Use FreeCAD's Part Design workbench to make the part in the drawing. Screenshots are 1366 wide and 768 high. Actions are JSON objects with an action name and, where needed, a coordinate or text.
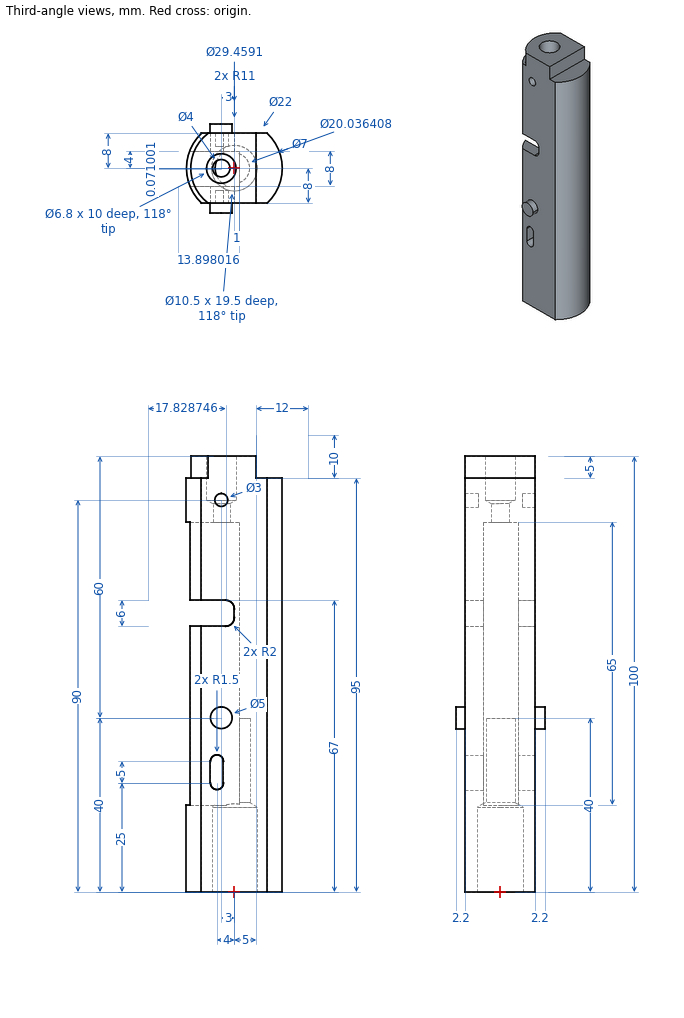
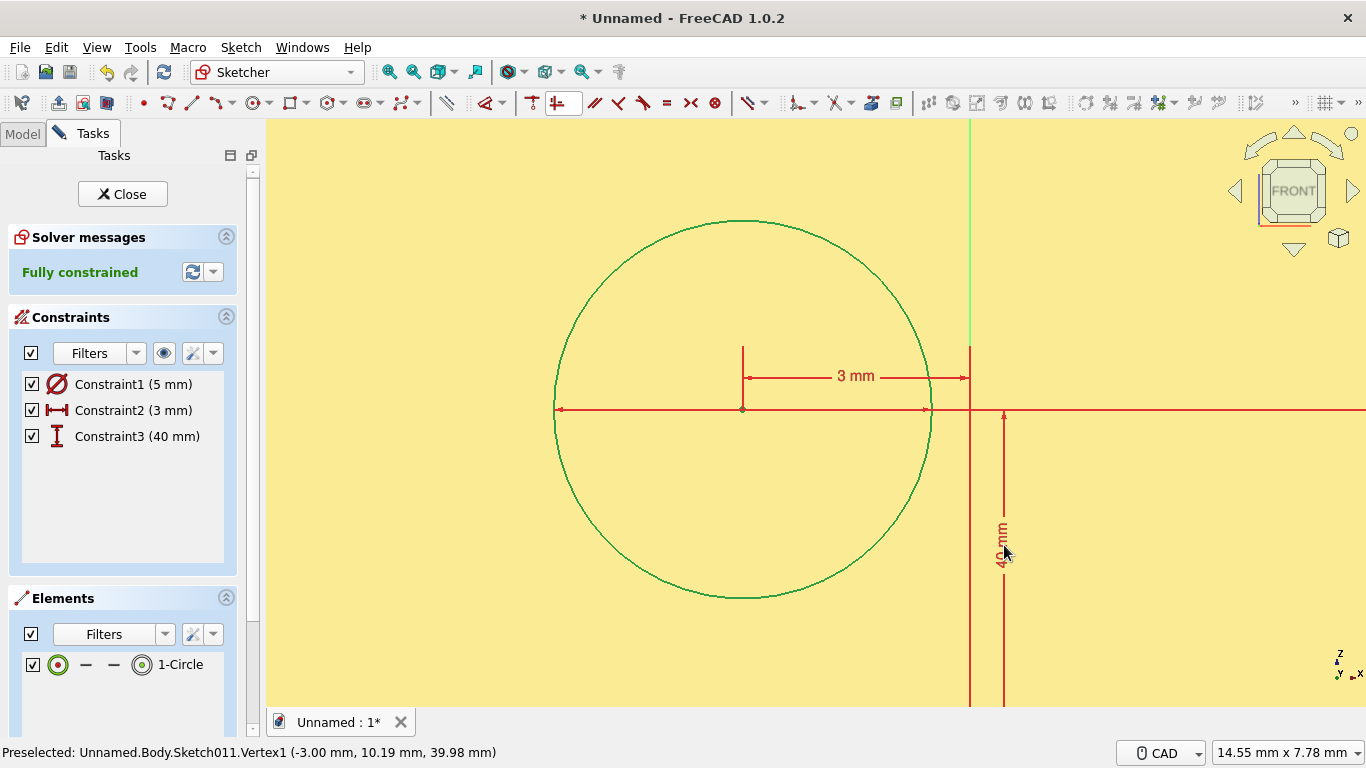
{"action": "left_click", "coordinate": [123, 194]}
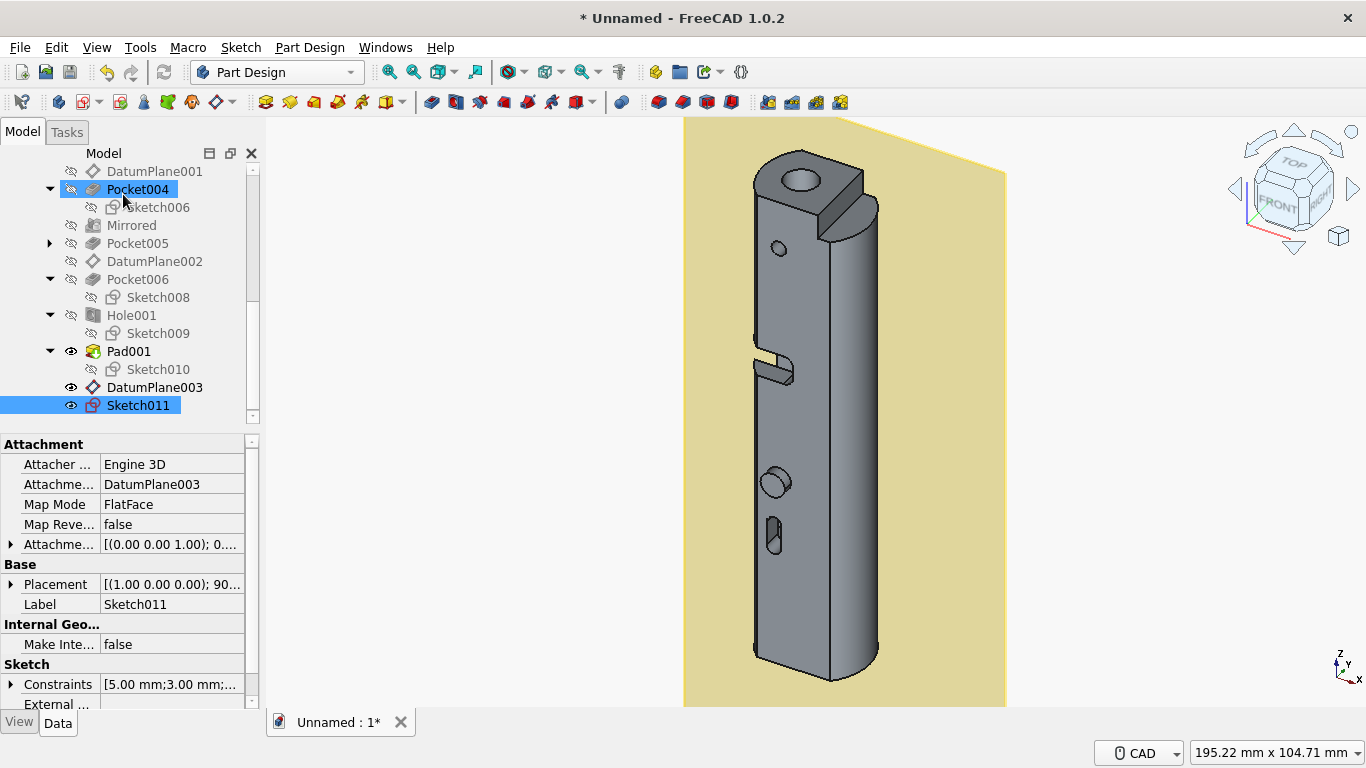
{"action": "left_click", "coordinate": [266, 102]}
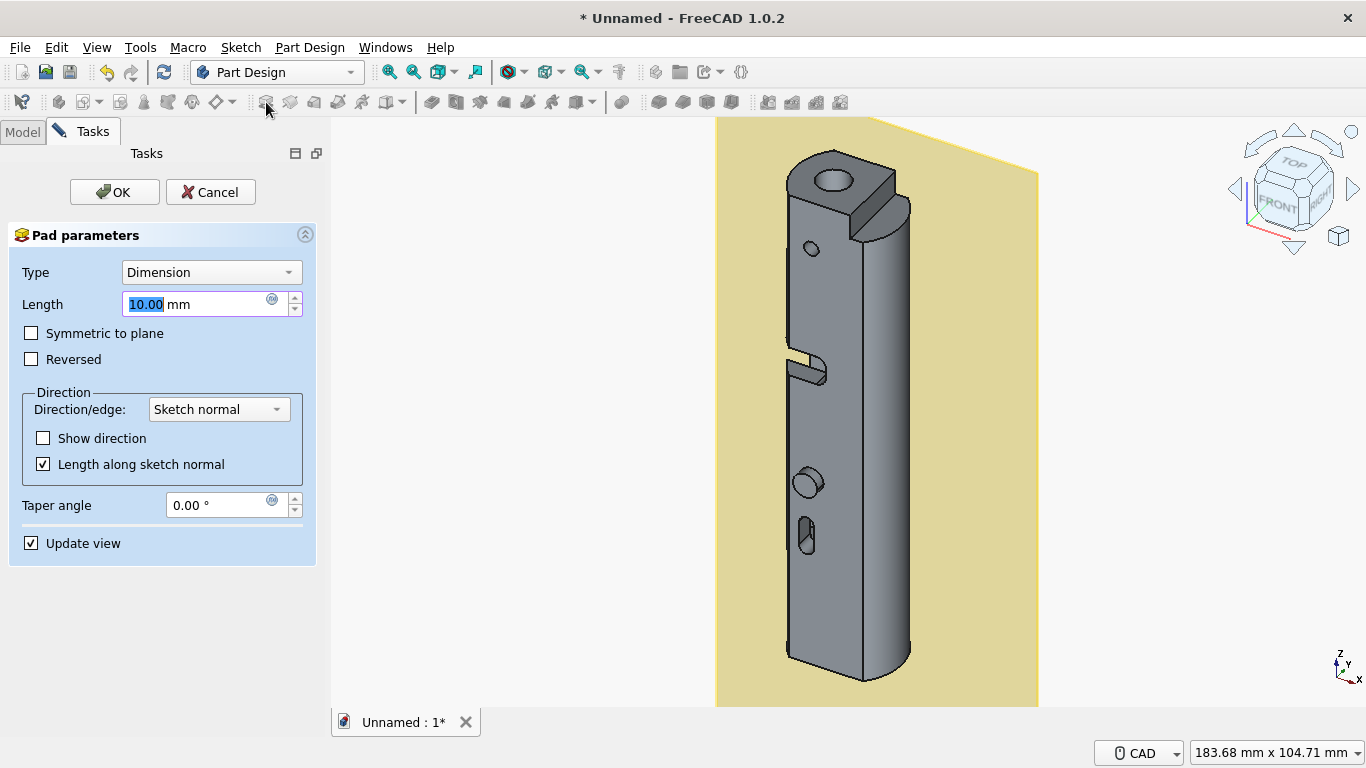
{"action": "type", "text": "2.2"}
{"action": "key", "text": "Tab"}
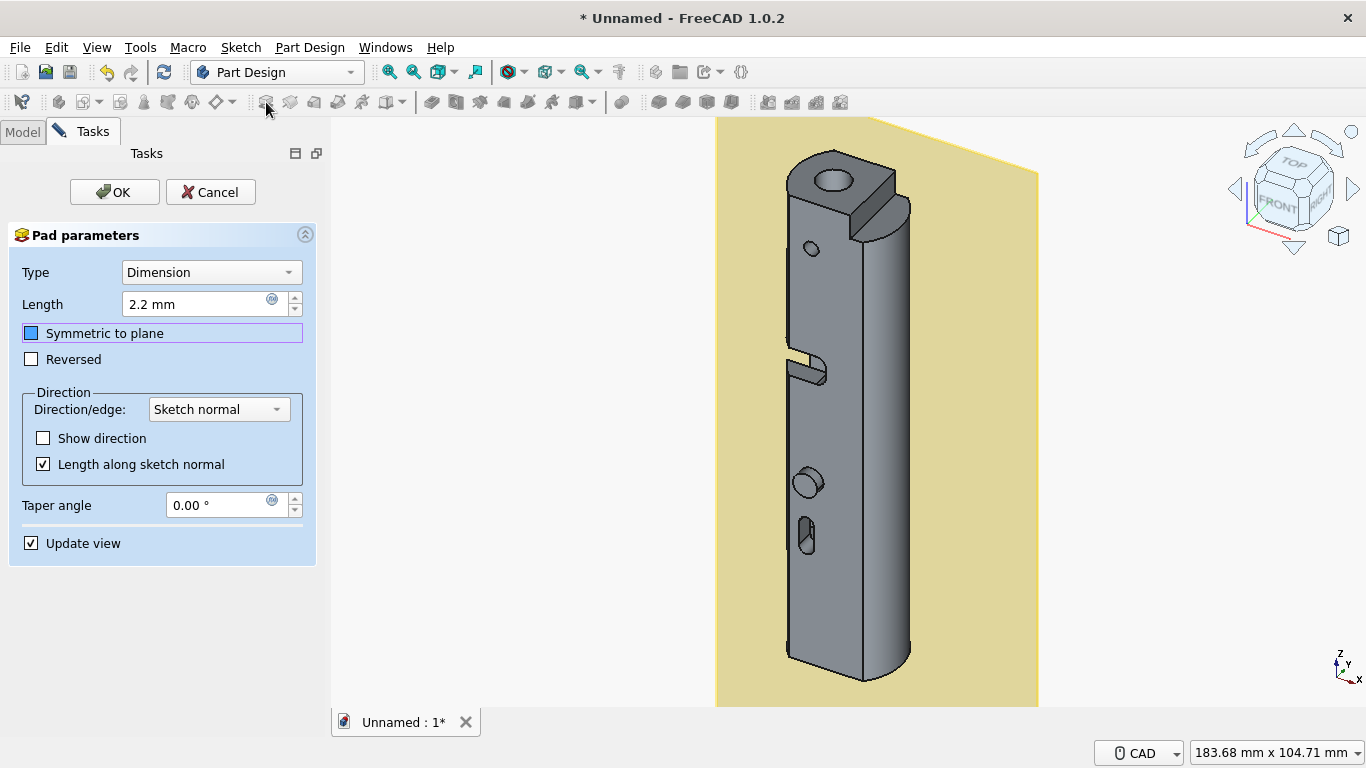
{"action": "left_click", "coordinate": [115, 192]}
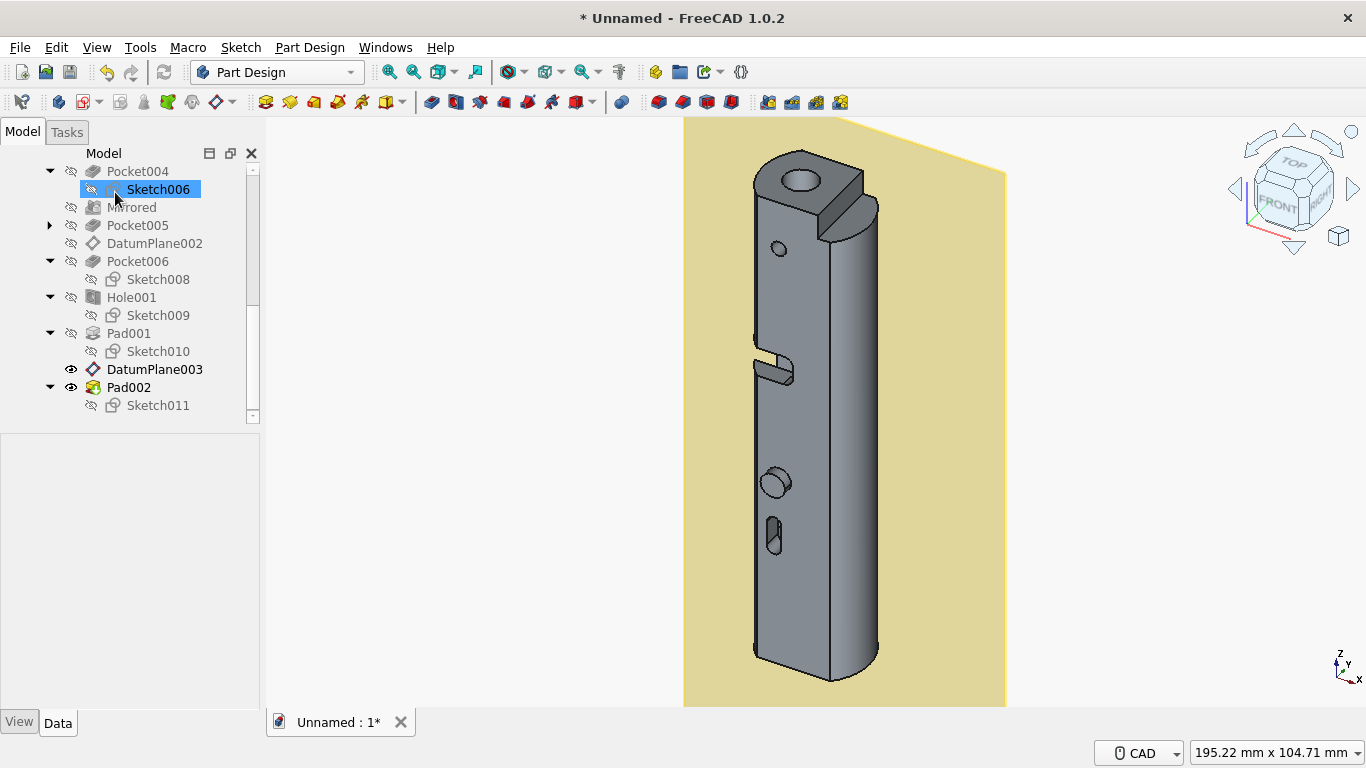
{"action": "left_click", "coordinate": [116, 369]}
{"action": "key", "text": "space"}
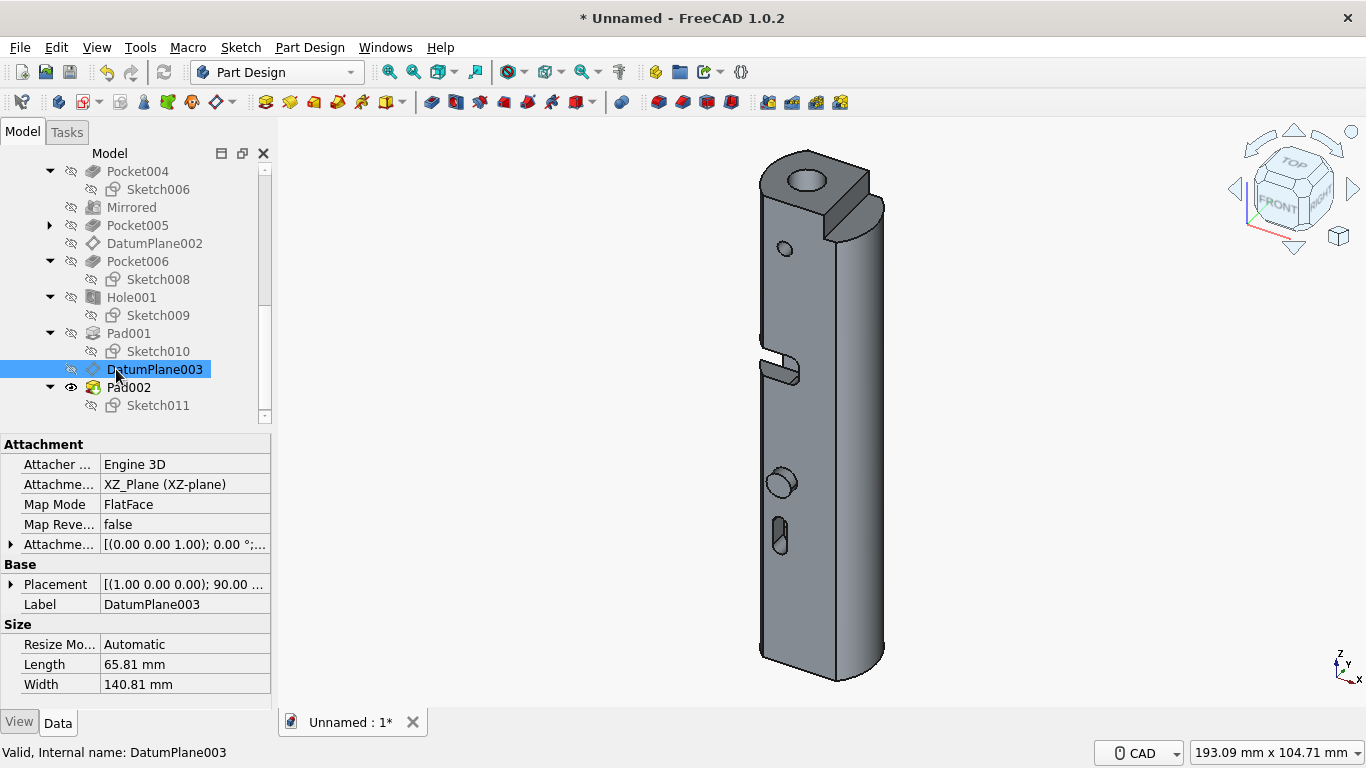
{"action": "left_click", "coordinate": [318, 667]}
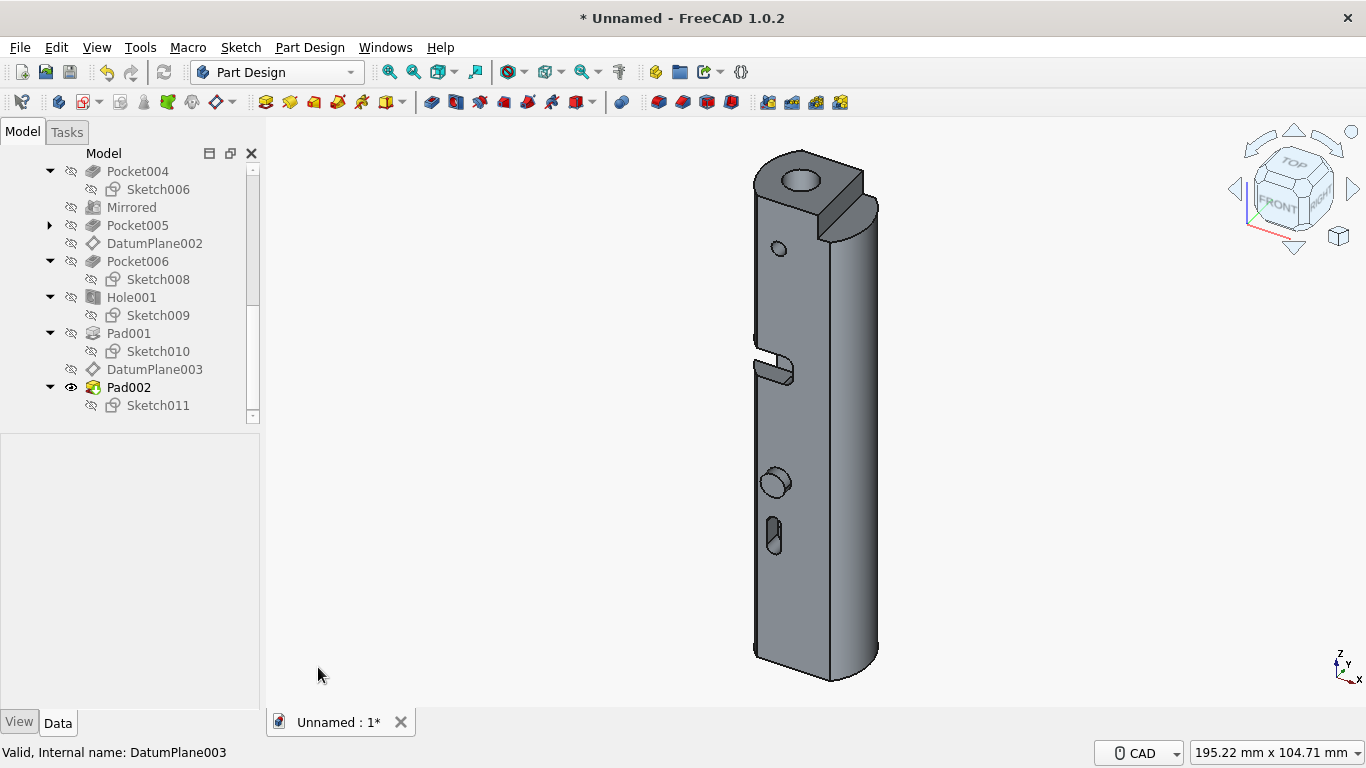
{"action": "left_click", "coordinate": [84, 102]}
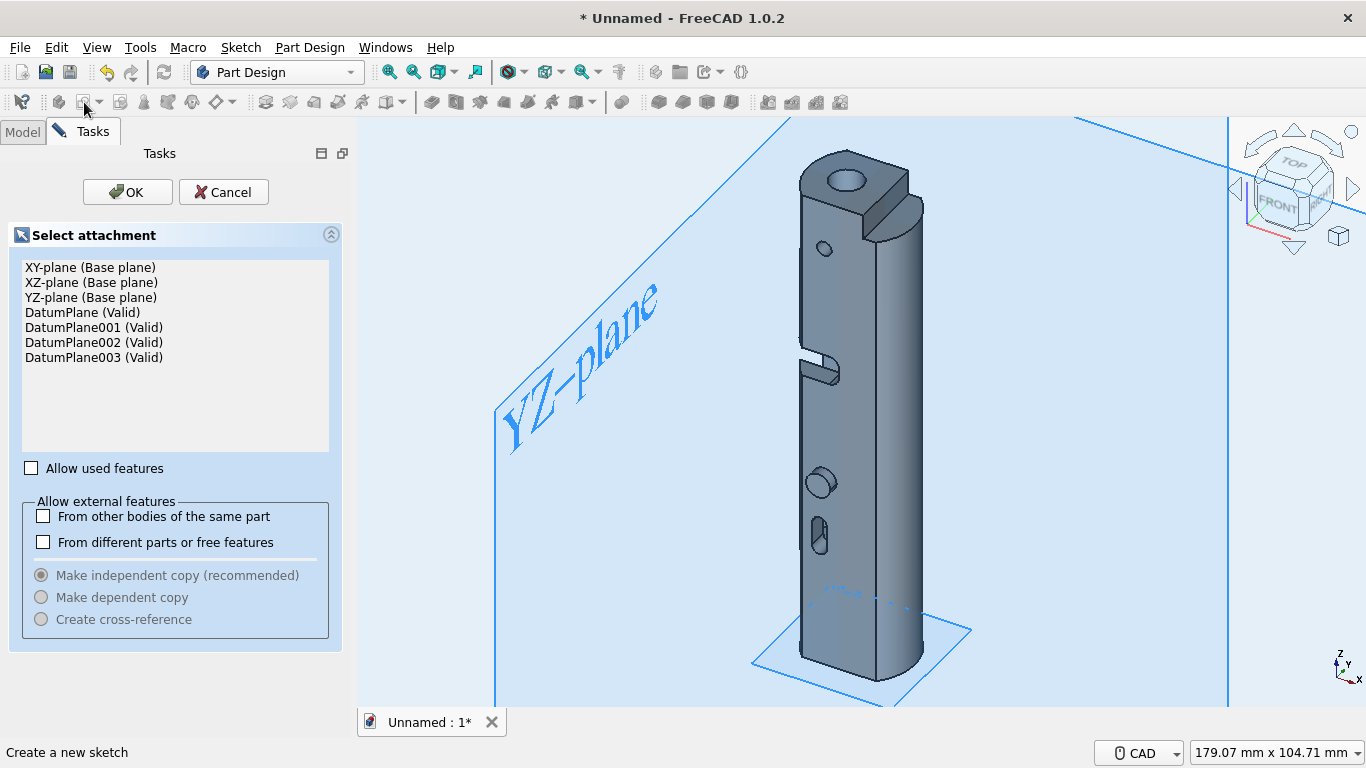
{"action": "left_click", "coordinate": [82, 268]}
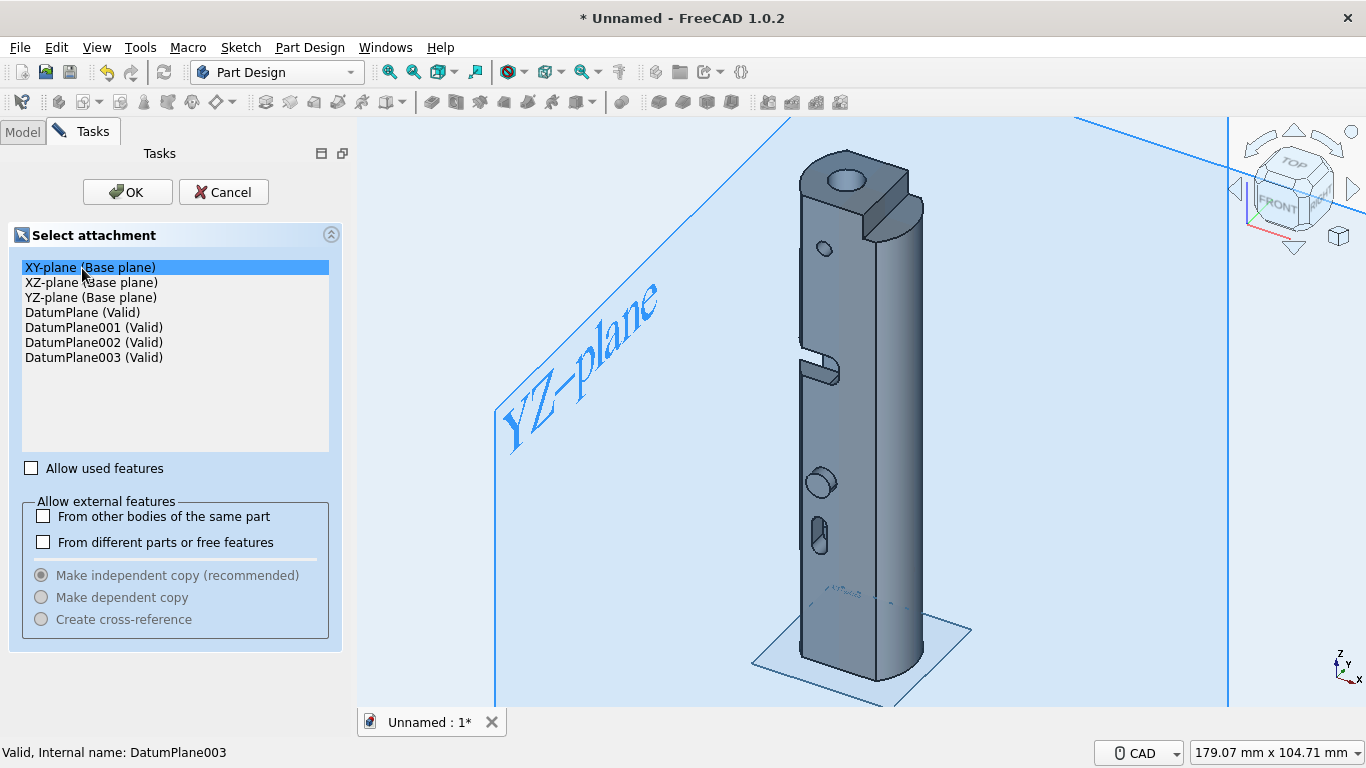
{"action": "left_click", "coordinate": [128, 192]}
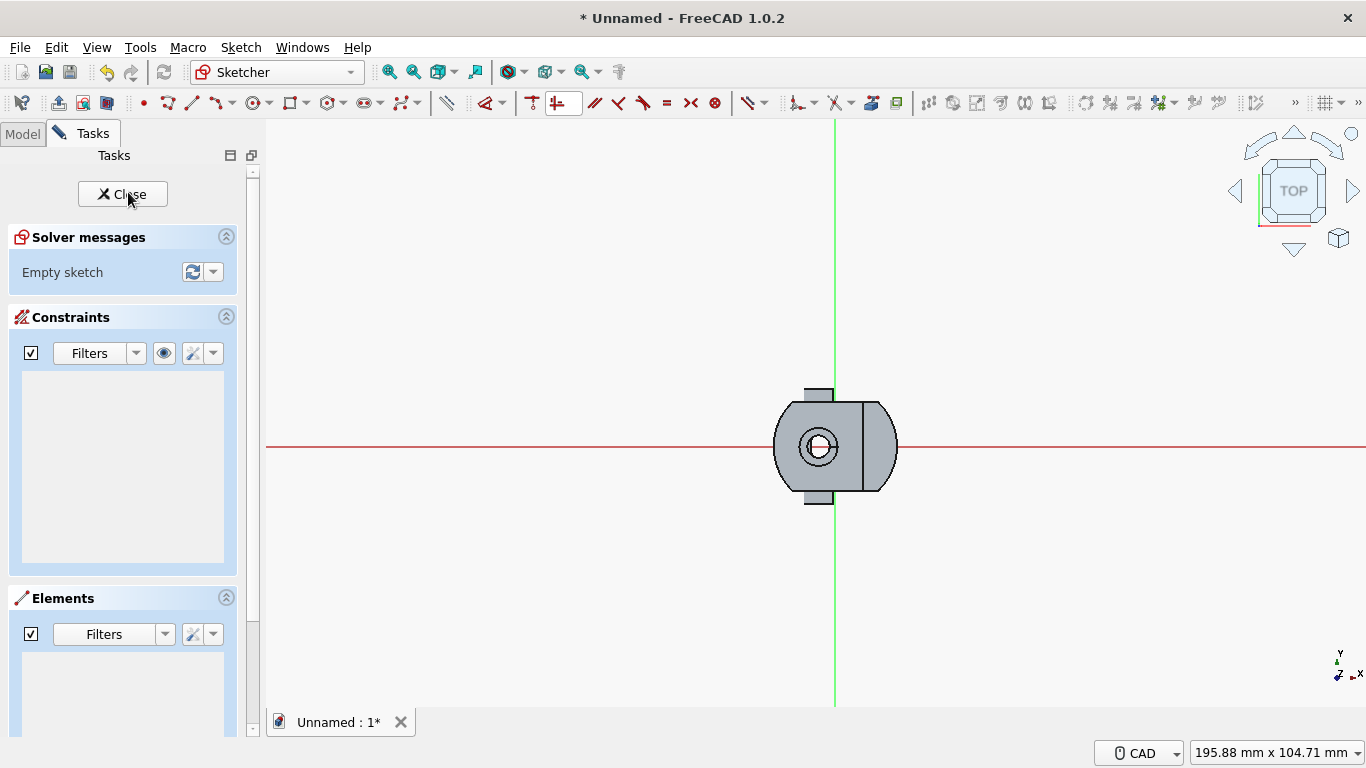
{"action": "key", "text": "q s"}